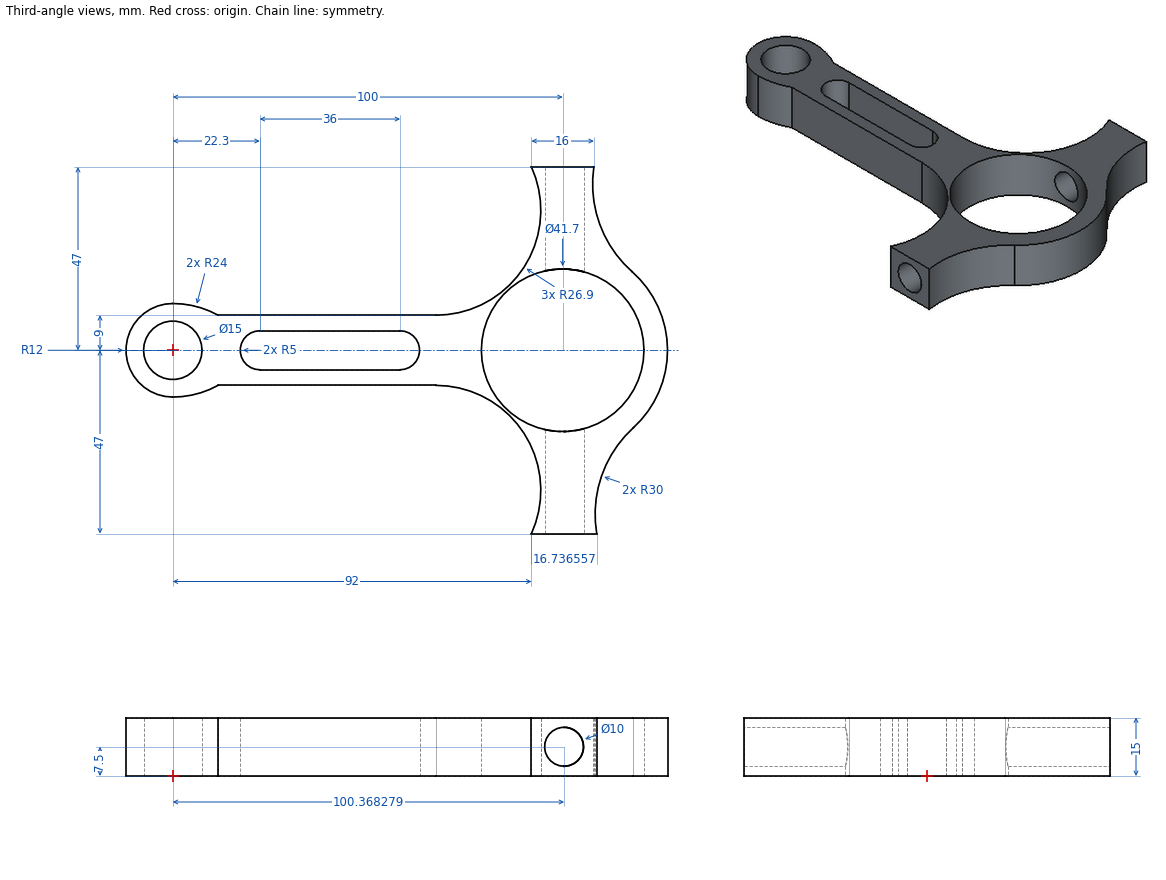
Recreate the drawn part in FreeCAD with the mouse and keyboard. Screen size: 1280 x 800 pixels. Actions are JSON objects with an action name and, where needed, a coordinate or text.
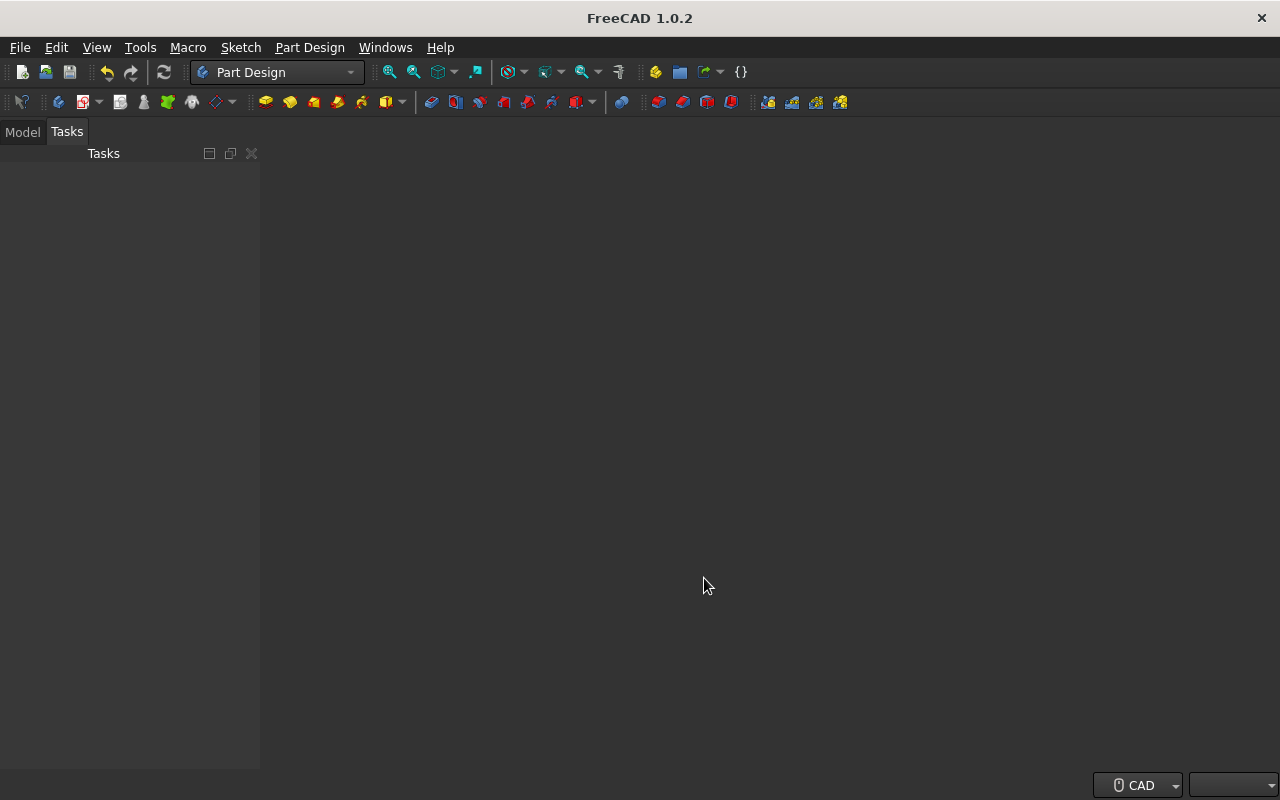
{"action": "left_click", "coordinate": [22, 72]}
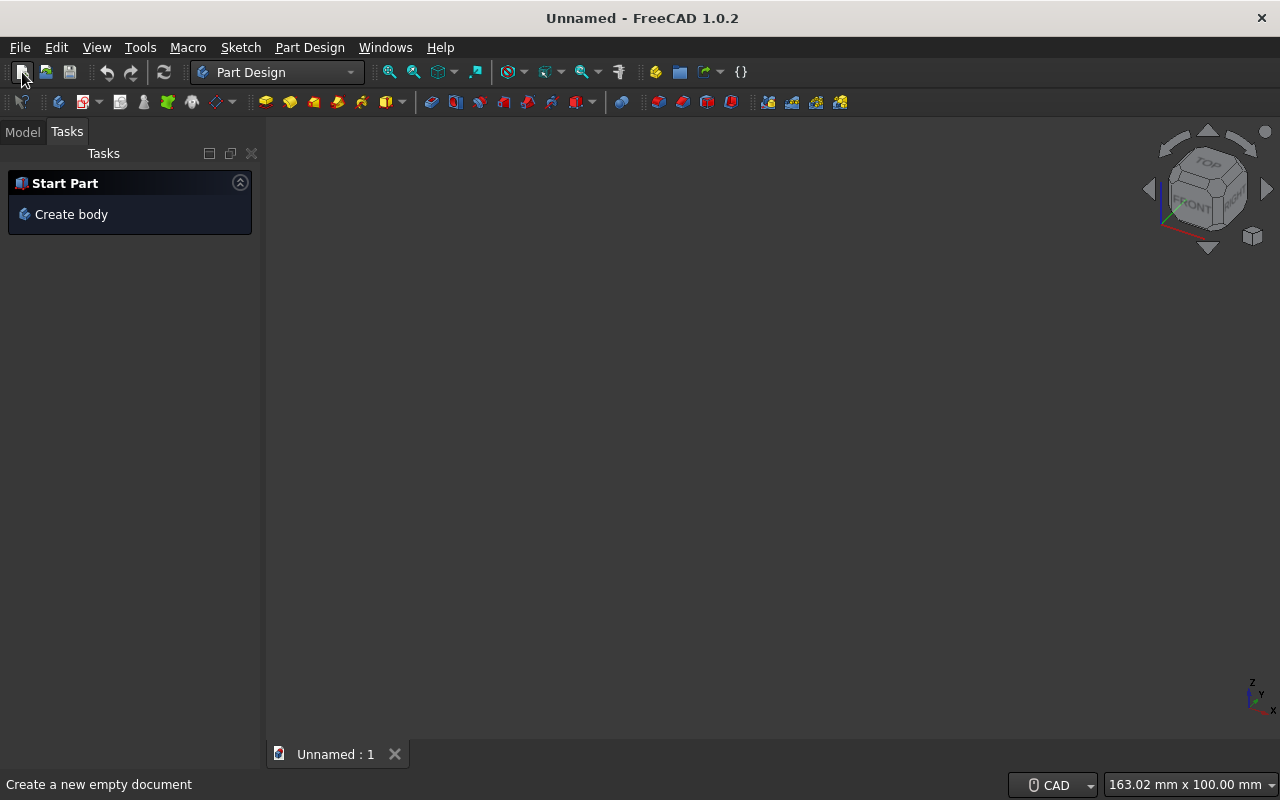
{"action": "left_click", "coordinate": [84, 102]}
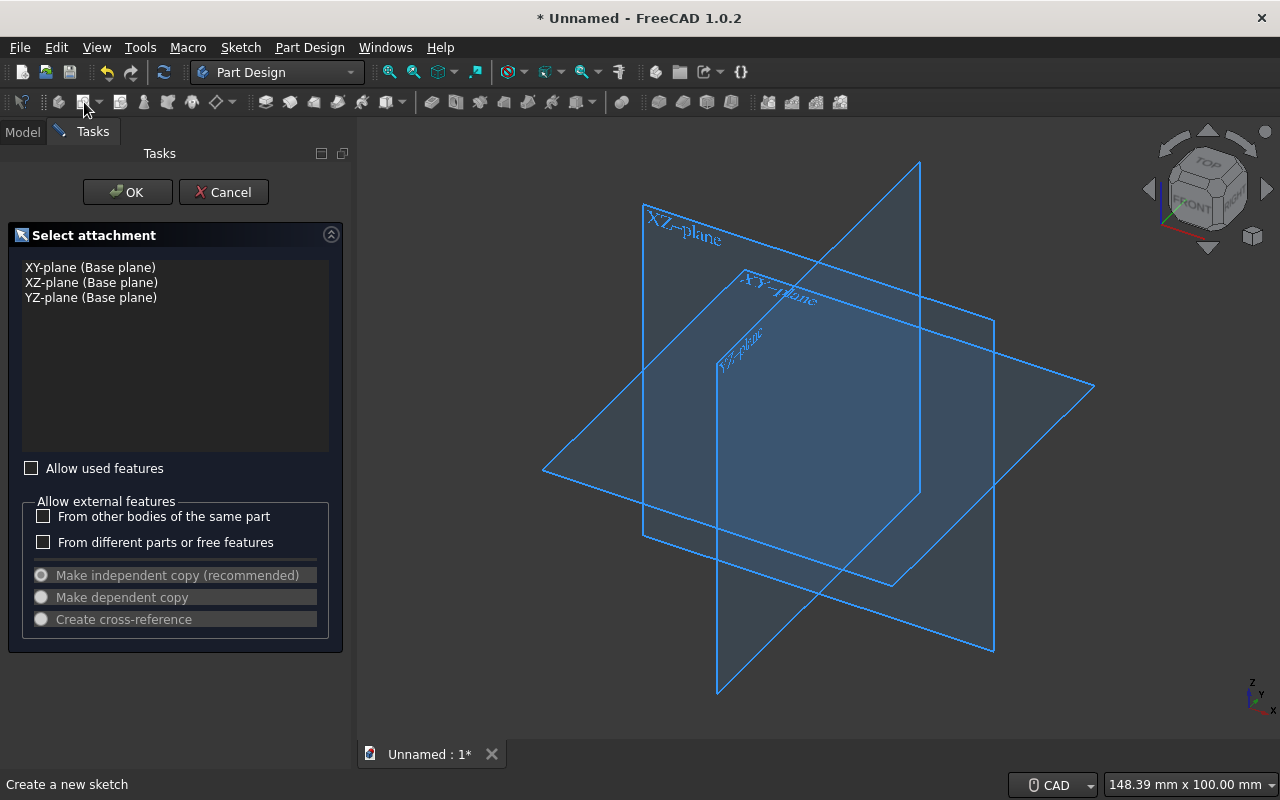
{"action": "left_click", "coordinate": [82, 268]}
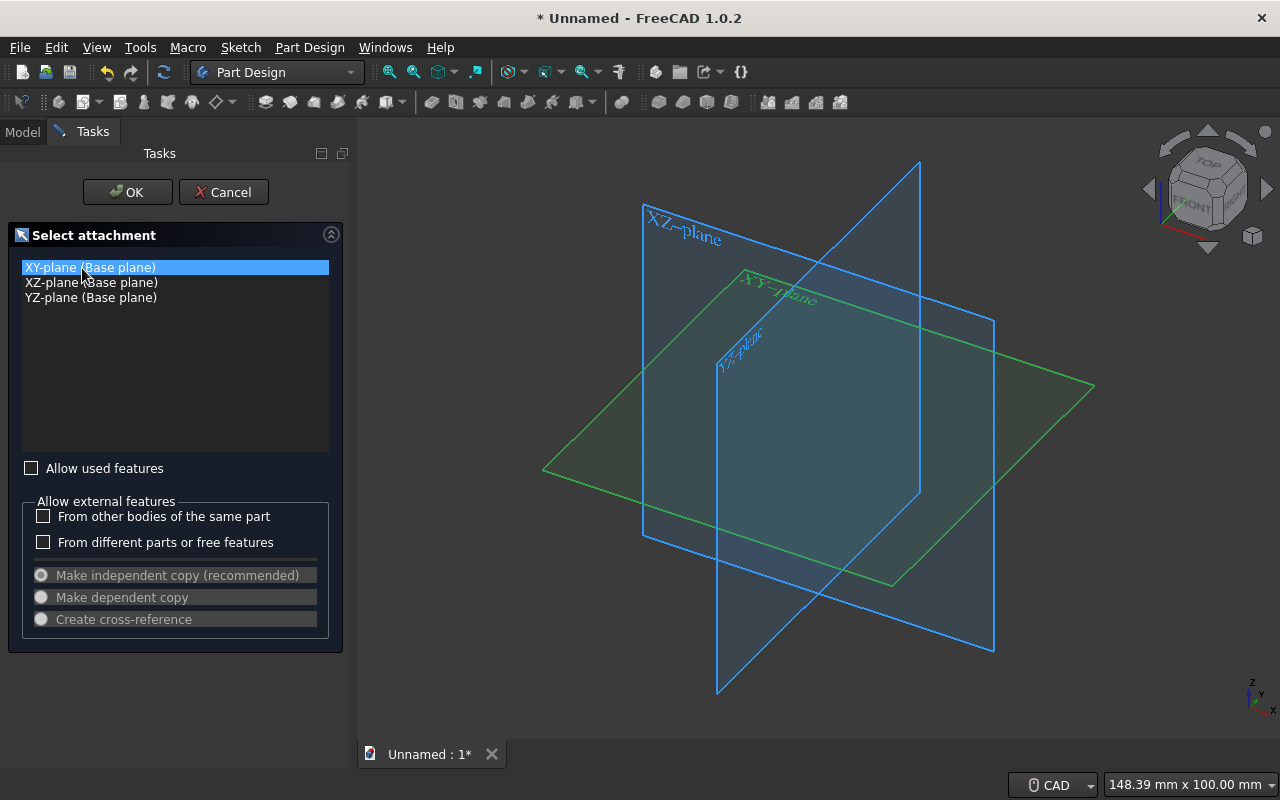
{"action": "left_click", "coordinate": [128, 192]}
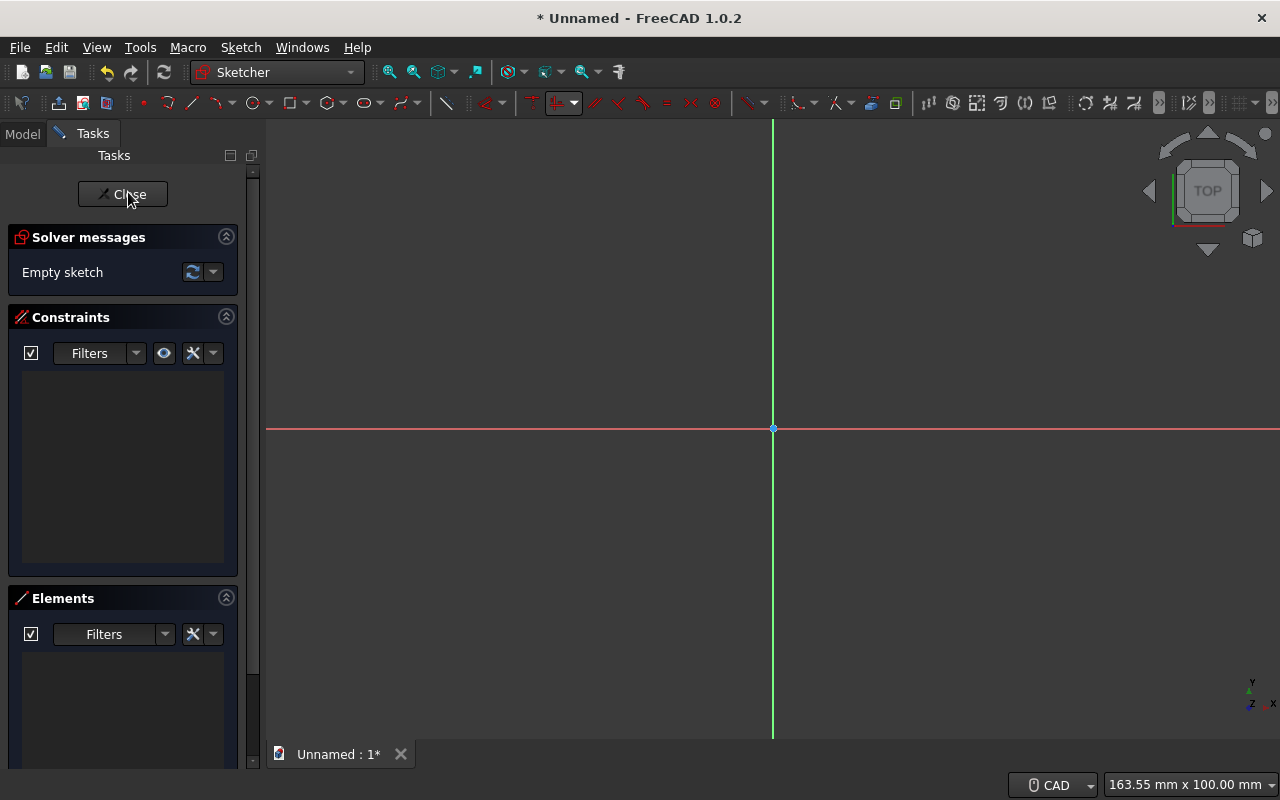
{"action": "scroll", "coordinate": [294, 429], "scroll_direction": "down", "scroll_amount": 3}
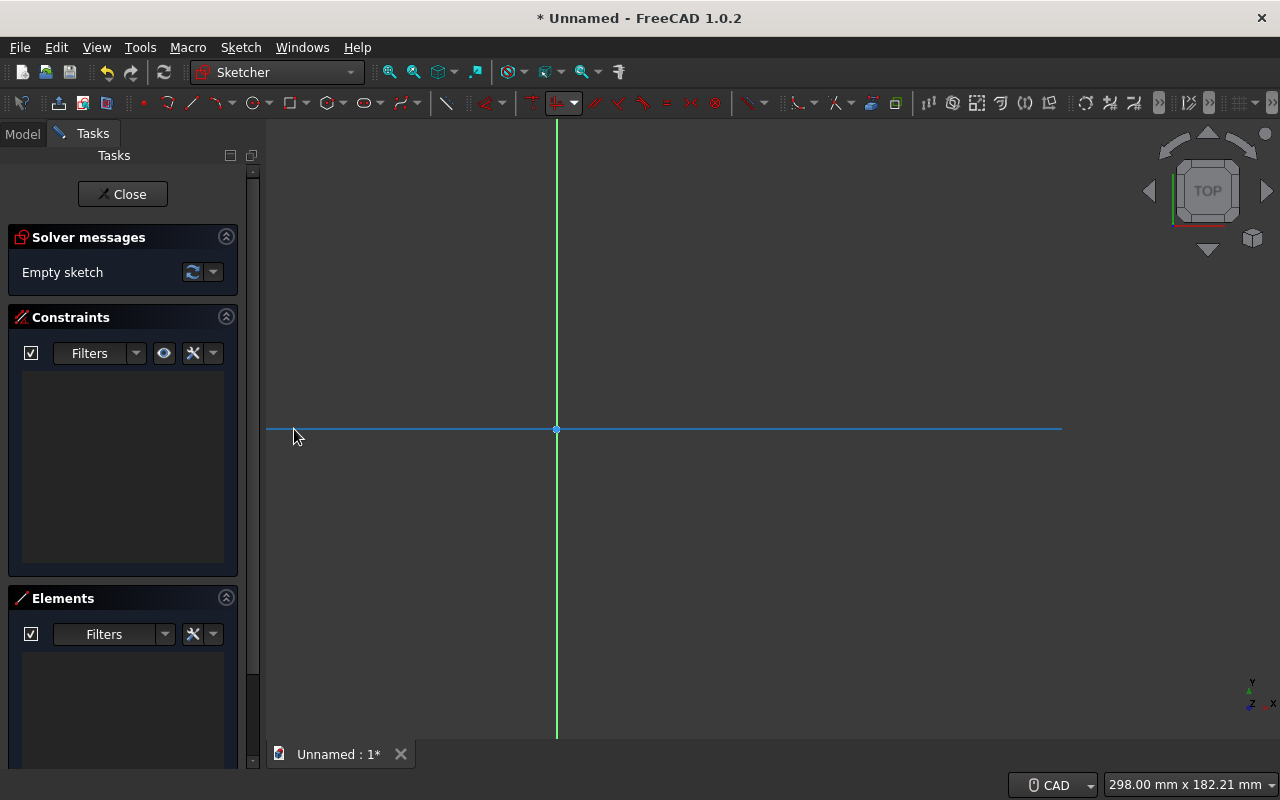
{"action": "left_click", "coordinate": [192, 104]}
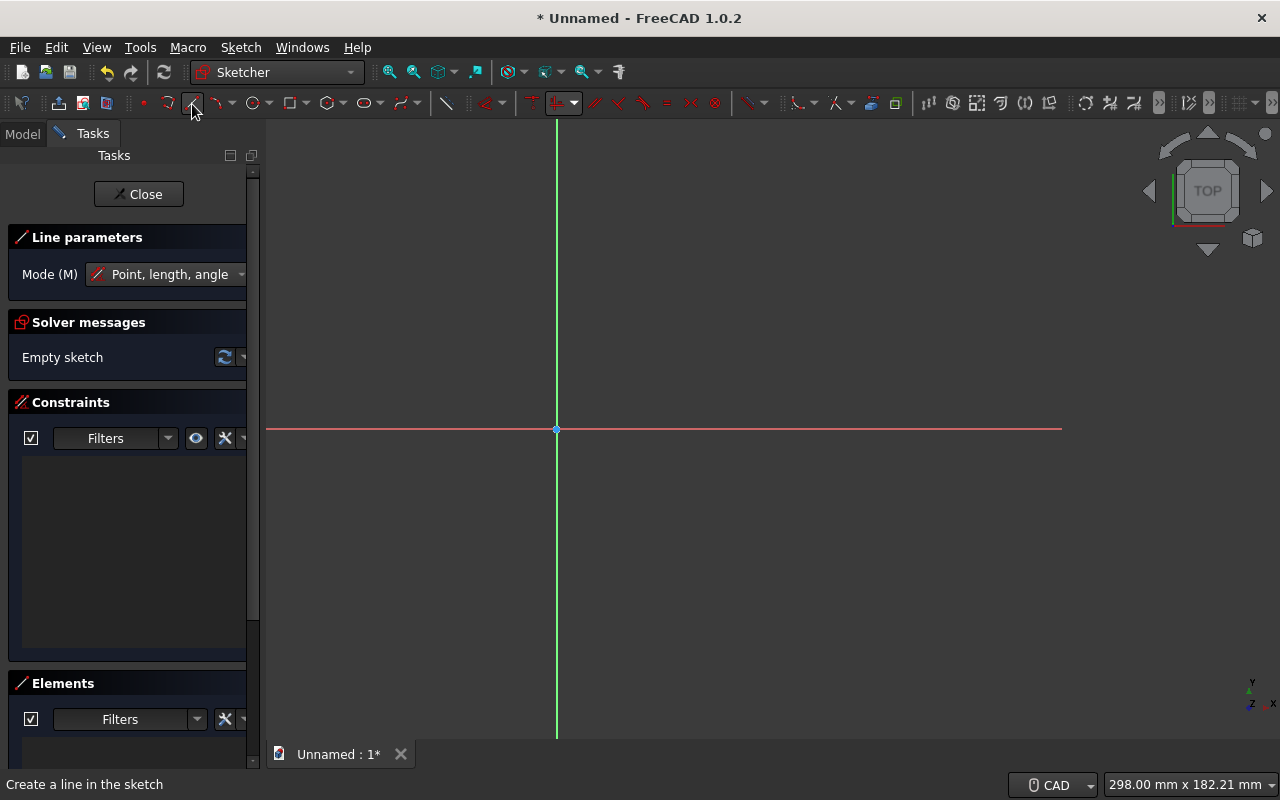
{"action": "left_click", "coordinate": [787, 399]}
{"action": "left_click", "coordinate": [596, 399]}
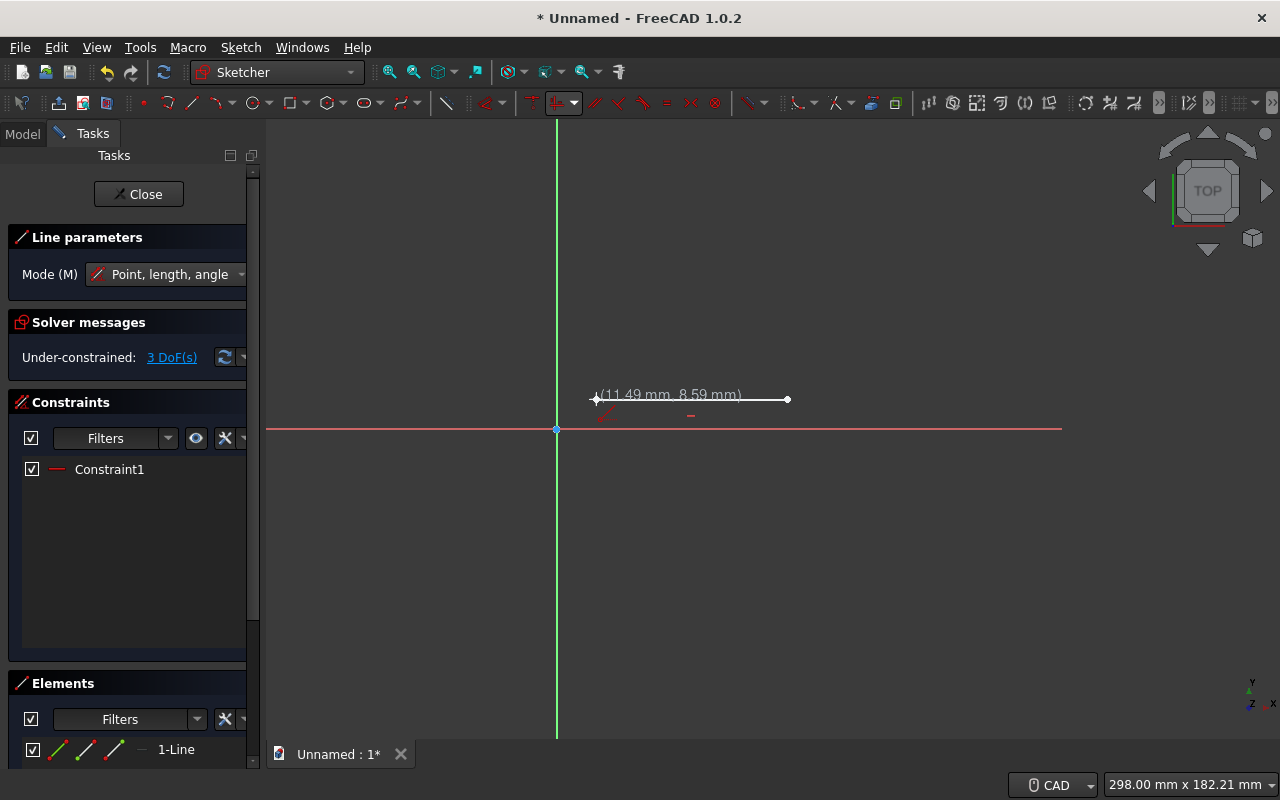
{"action": "left_click", "coordinate": [596, 460]}
{"action": "left_click", "coordinate": [787, 460]}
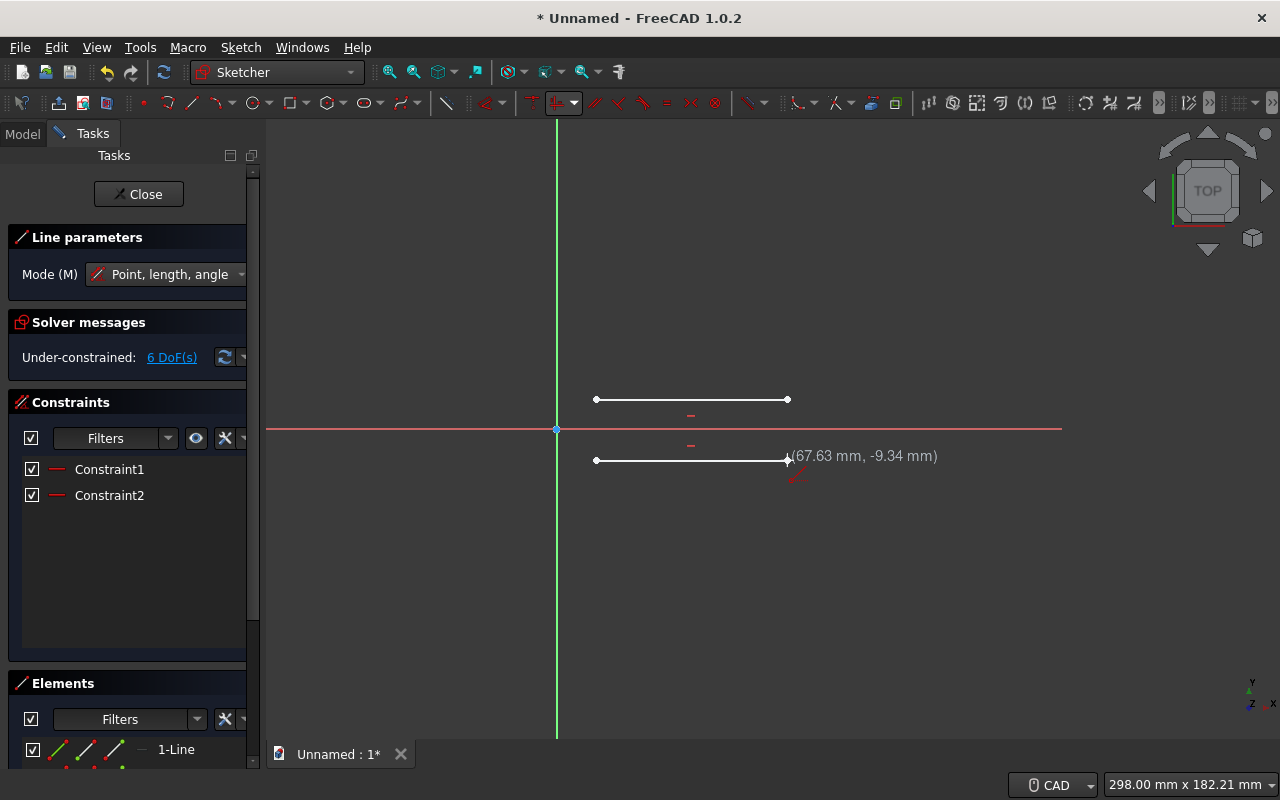
{"action": "left_click", "coordinate": [870, 589]}
{"action": "left_click", "coordinate": [927, 589]}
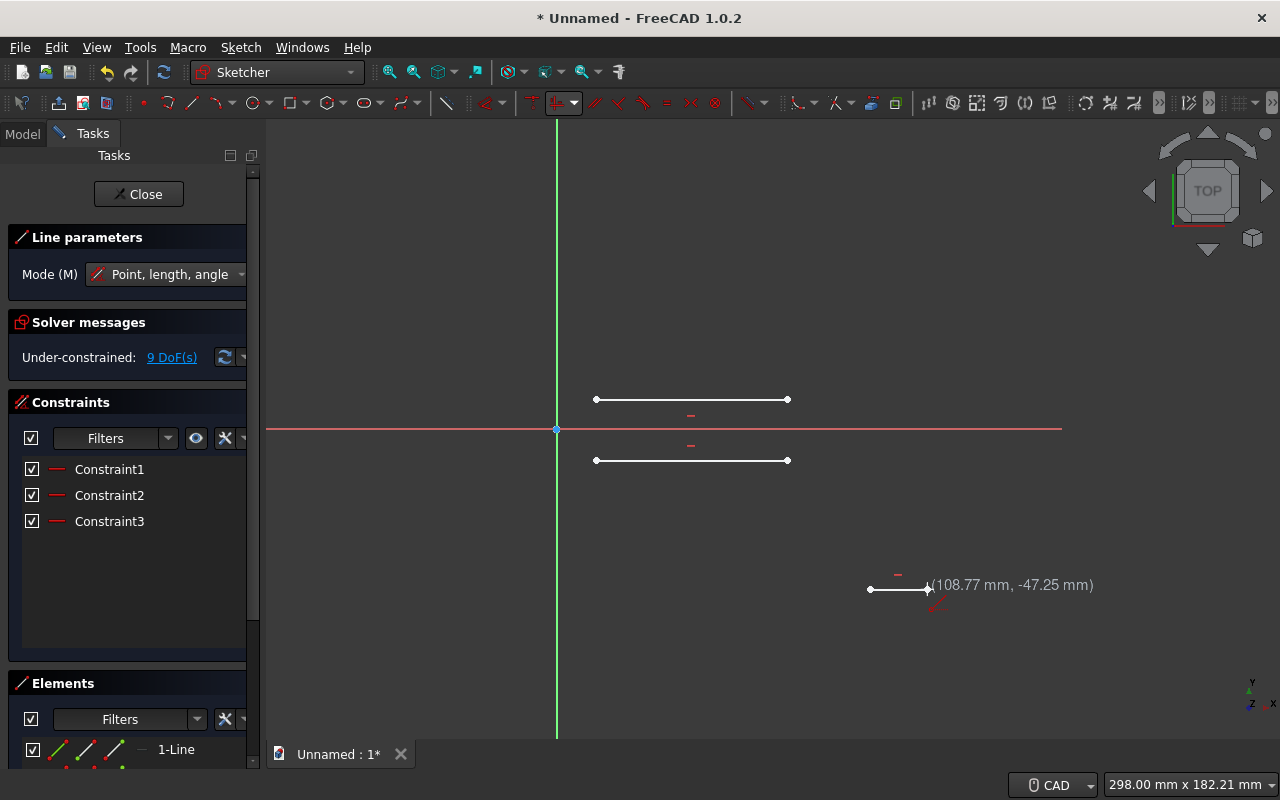
{"action": "left_click", "coordinate": [924, 269]}
{"action": "left_click", "coordinate": [870, 269]}